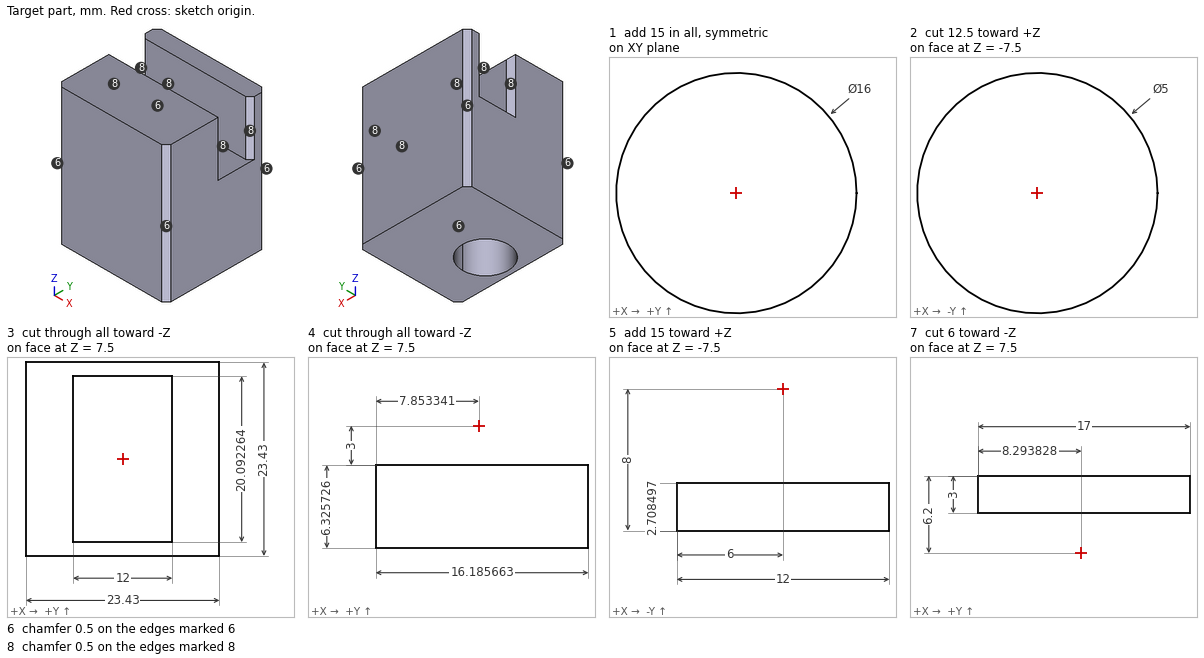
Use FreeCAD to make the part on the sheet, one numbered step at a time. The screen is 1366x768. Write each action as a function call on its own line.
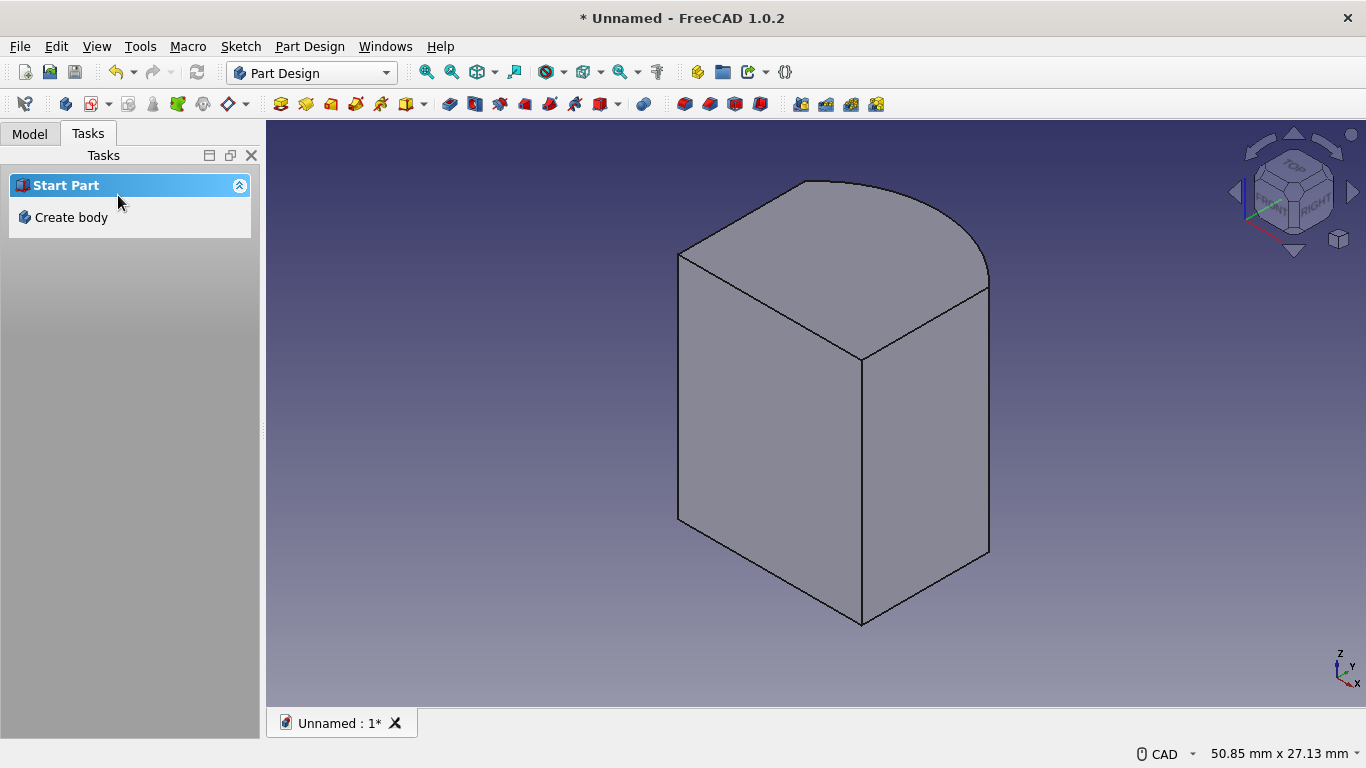
key(5)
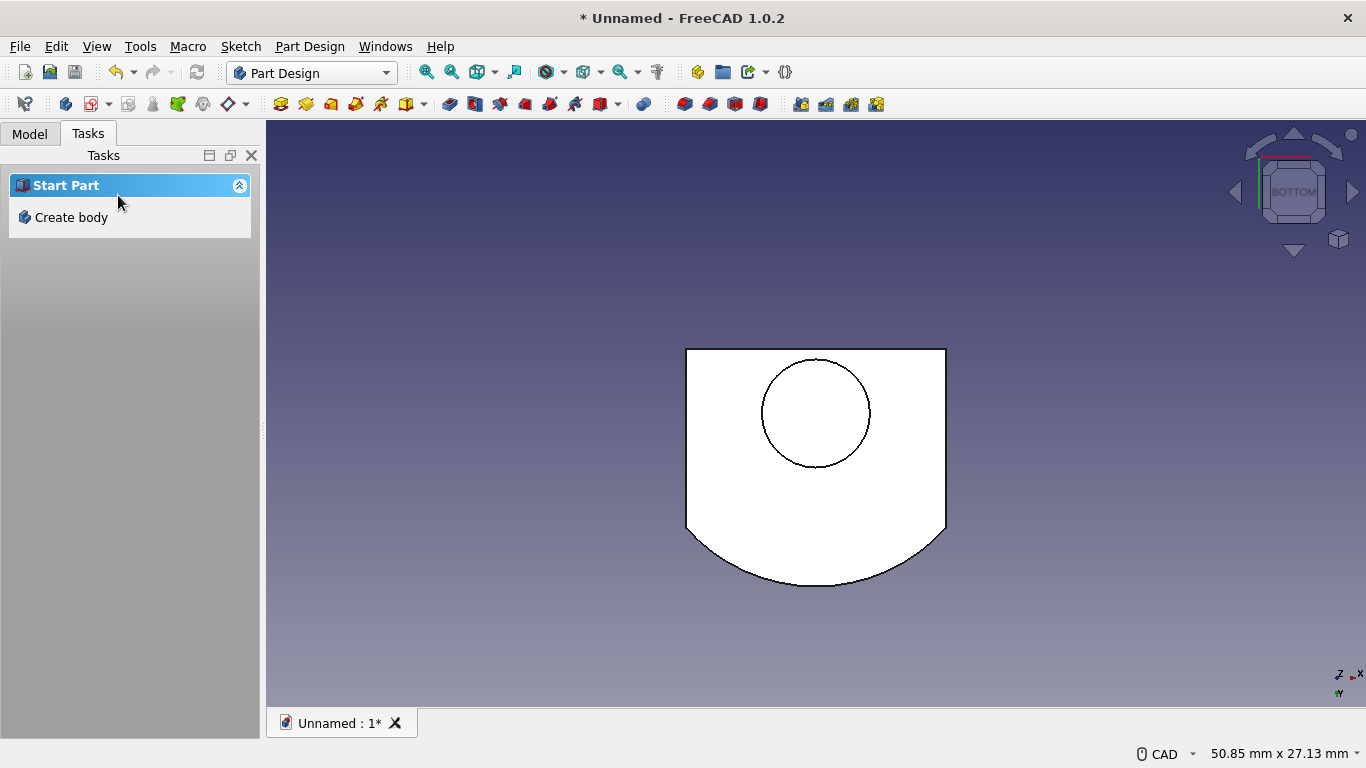
click(427, 72)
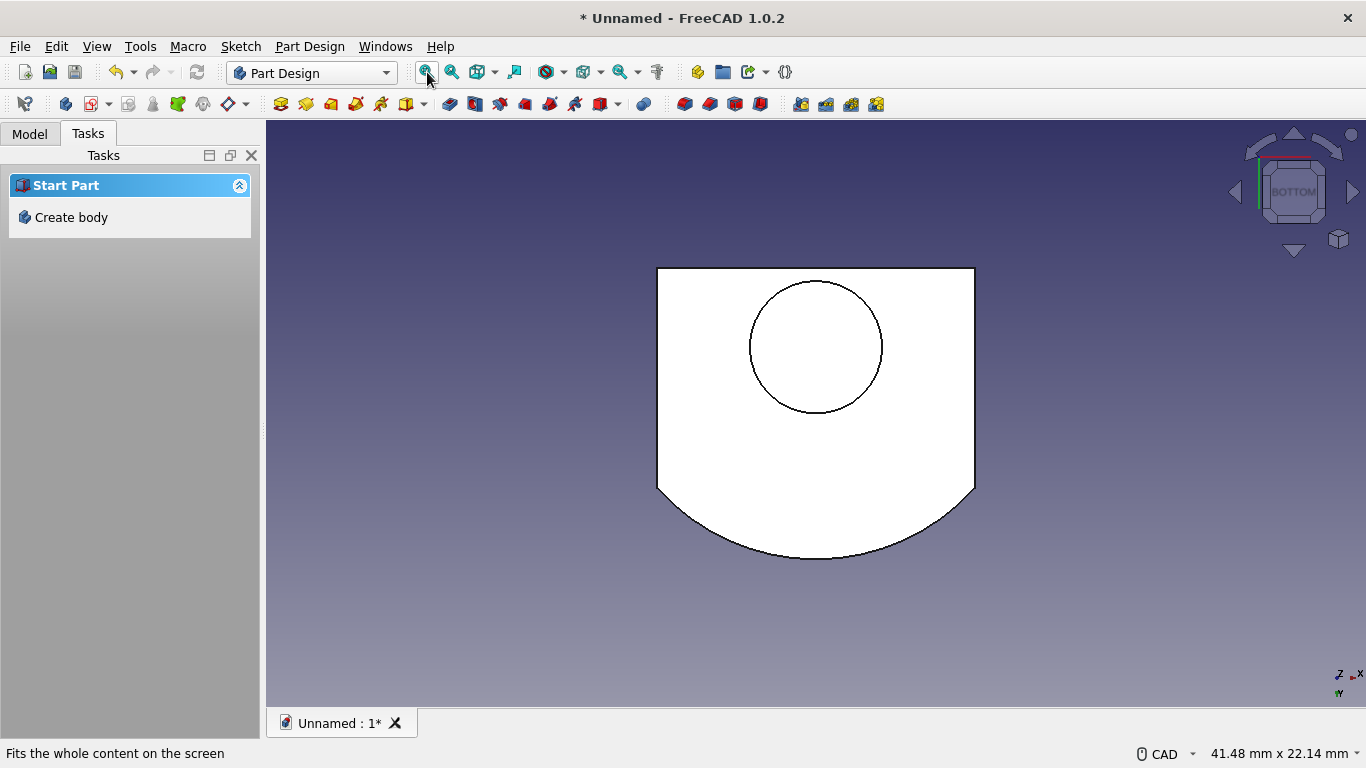
click(907, 454)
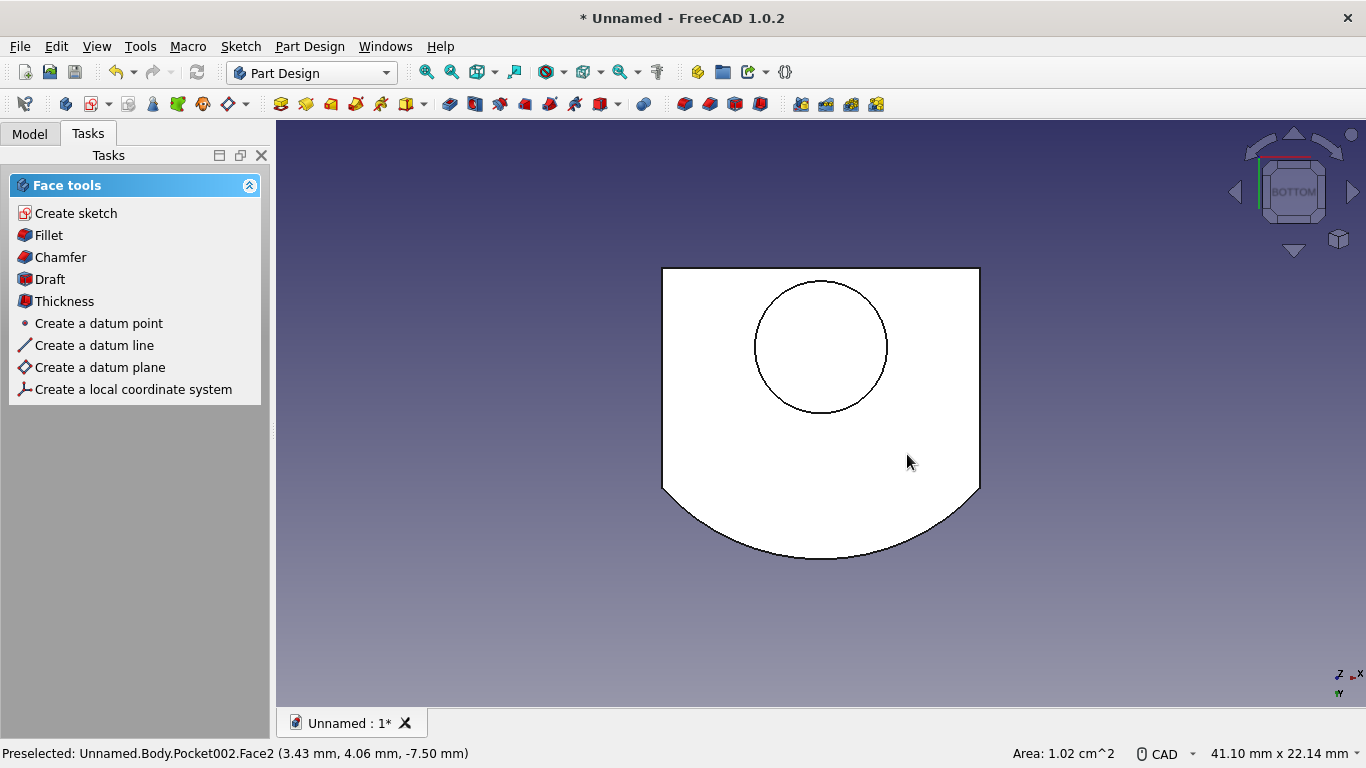
click(90, 104)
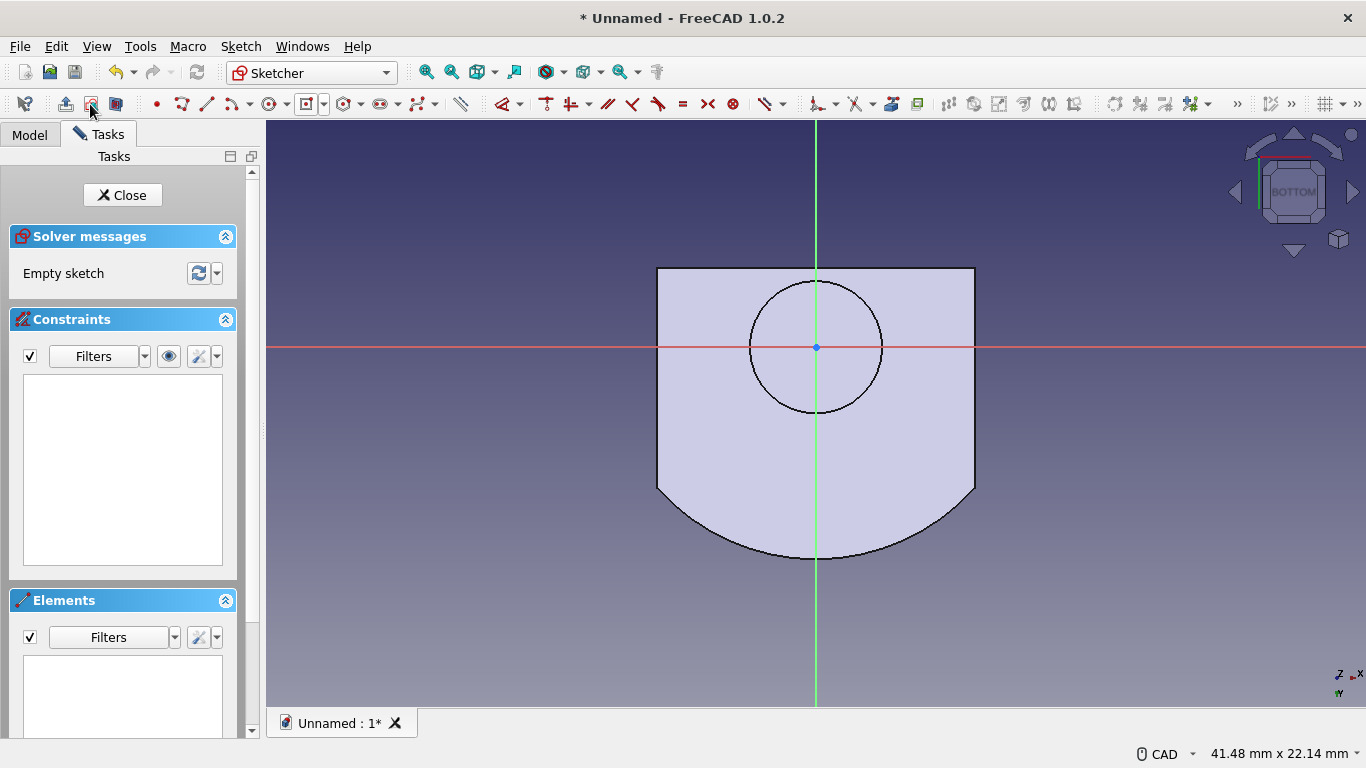
scroll(899, 502, up, 3)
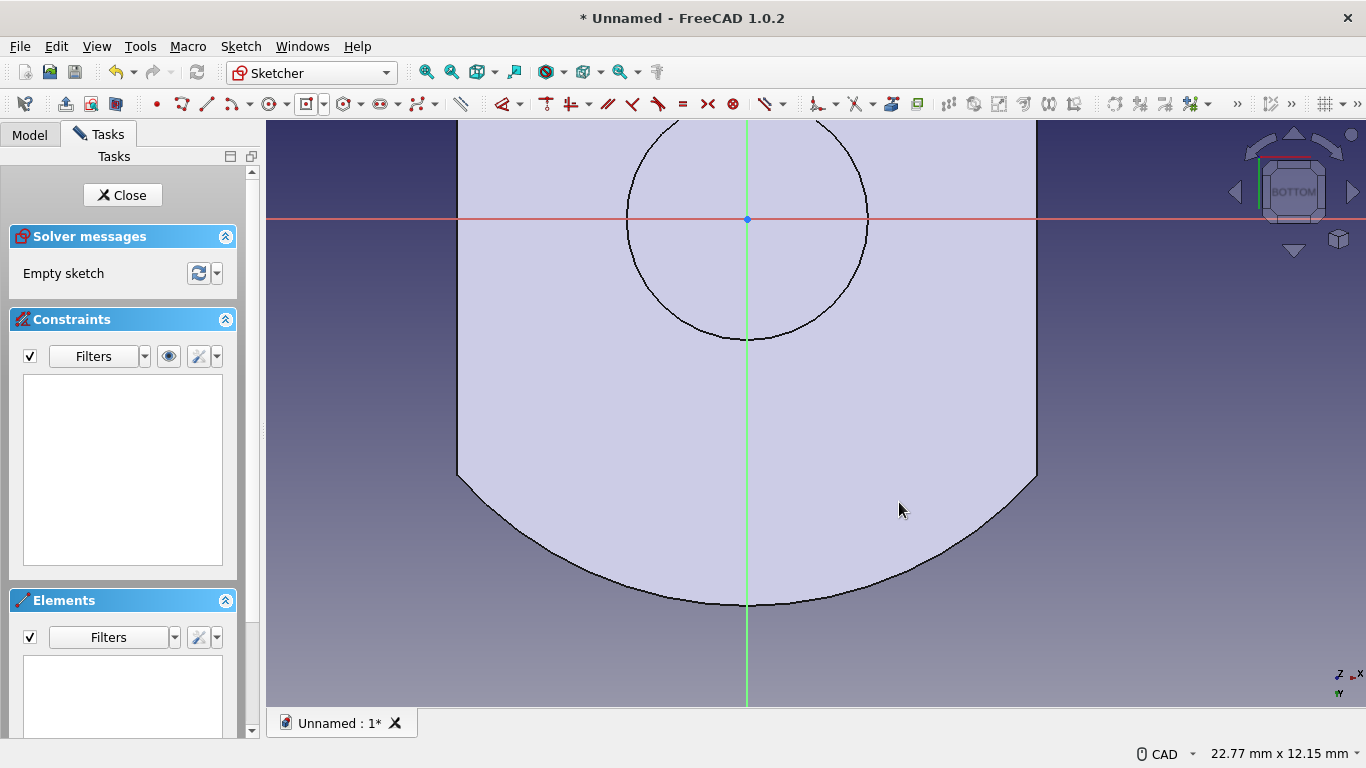
click(324, 104)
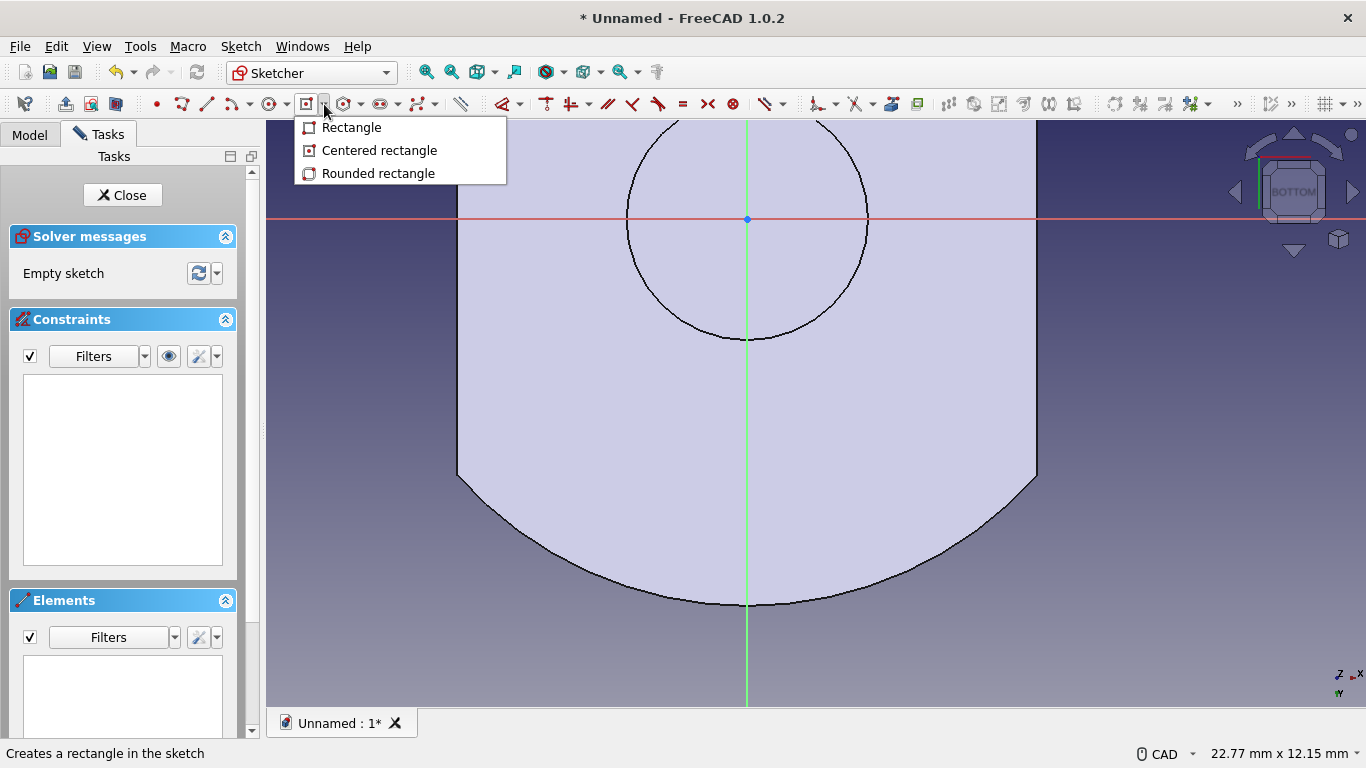
click(400, 128)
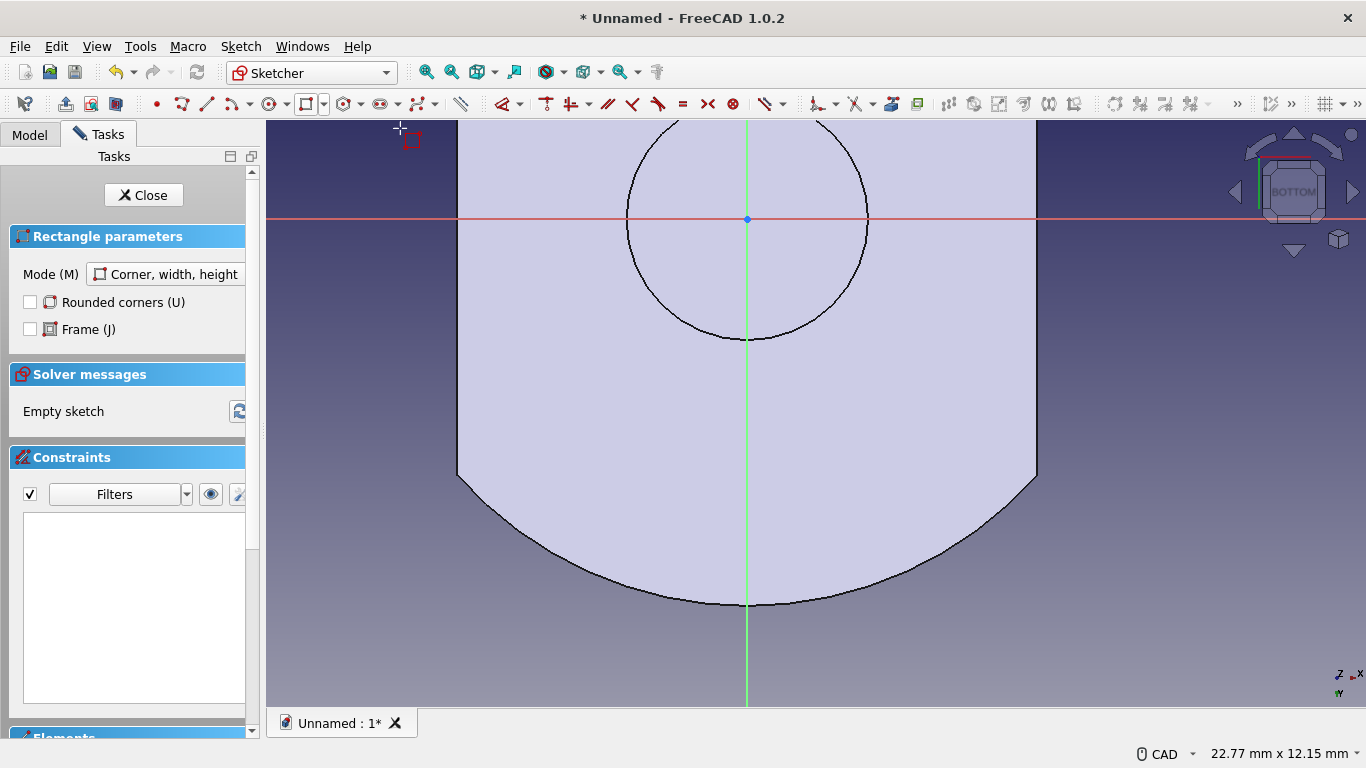
click(457, 475)
click(1037, 606)
key(Escape)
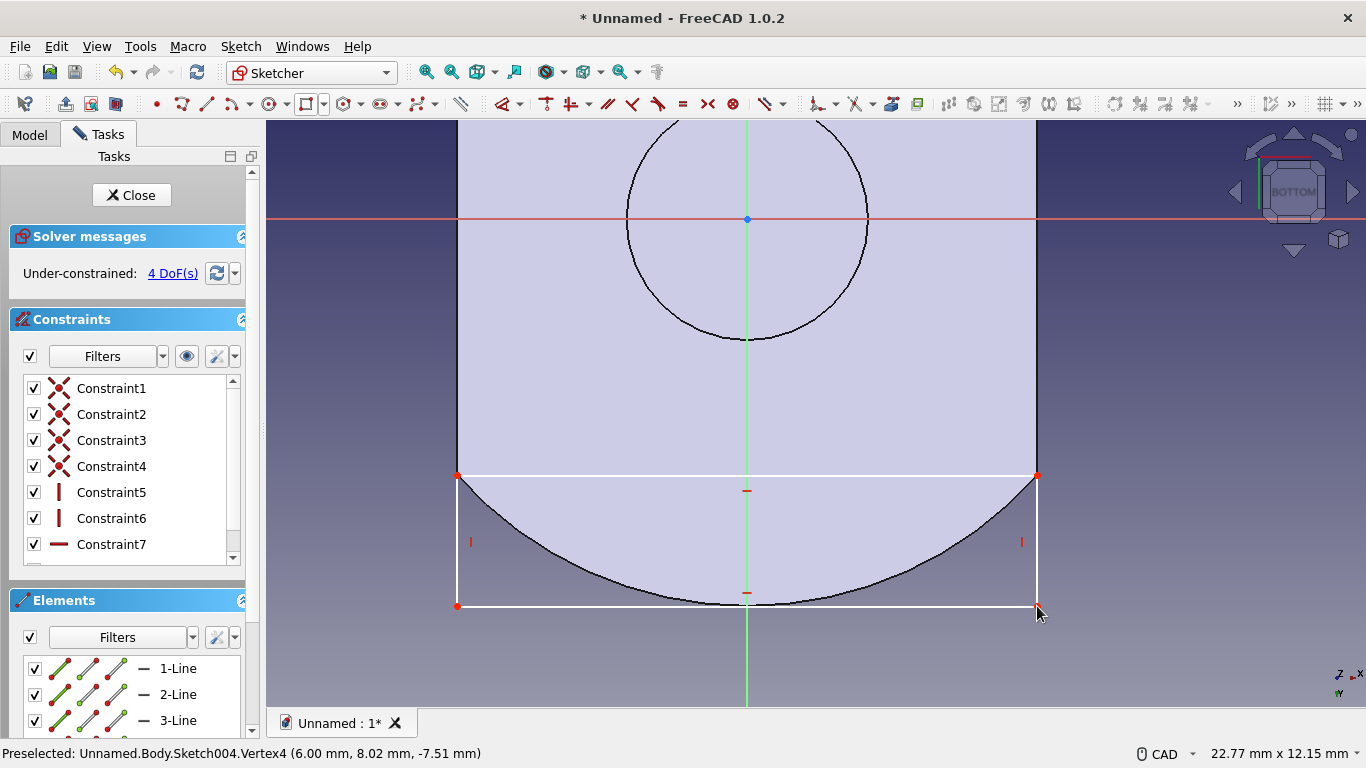
click(502, 104)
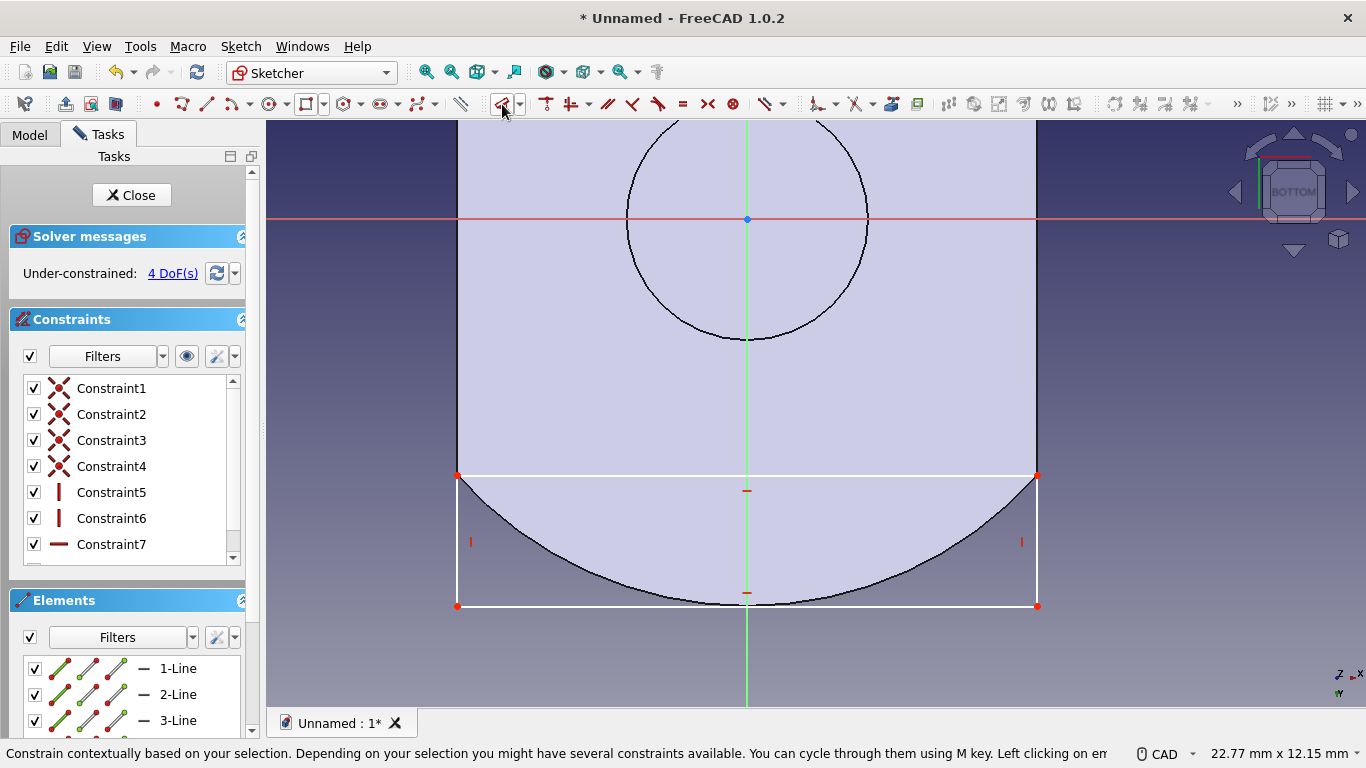
click(631, 607)
click(614, 641)